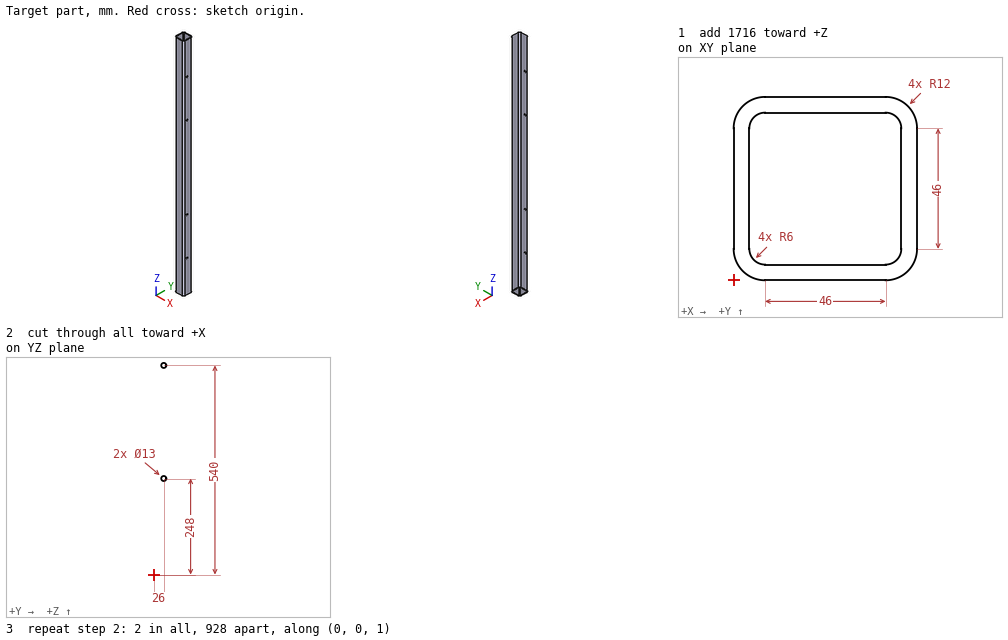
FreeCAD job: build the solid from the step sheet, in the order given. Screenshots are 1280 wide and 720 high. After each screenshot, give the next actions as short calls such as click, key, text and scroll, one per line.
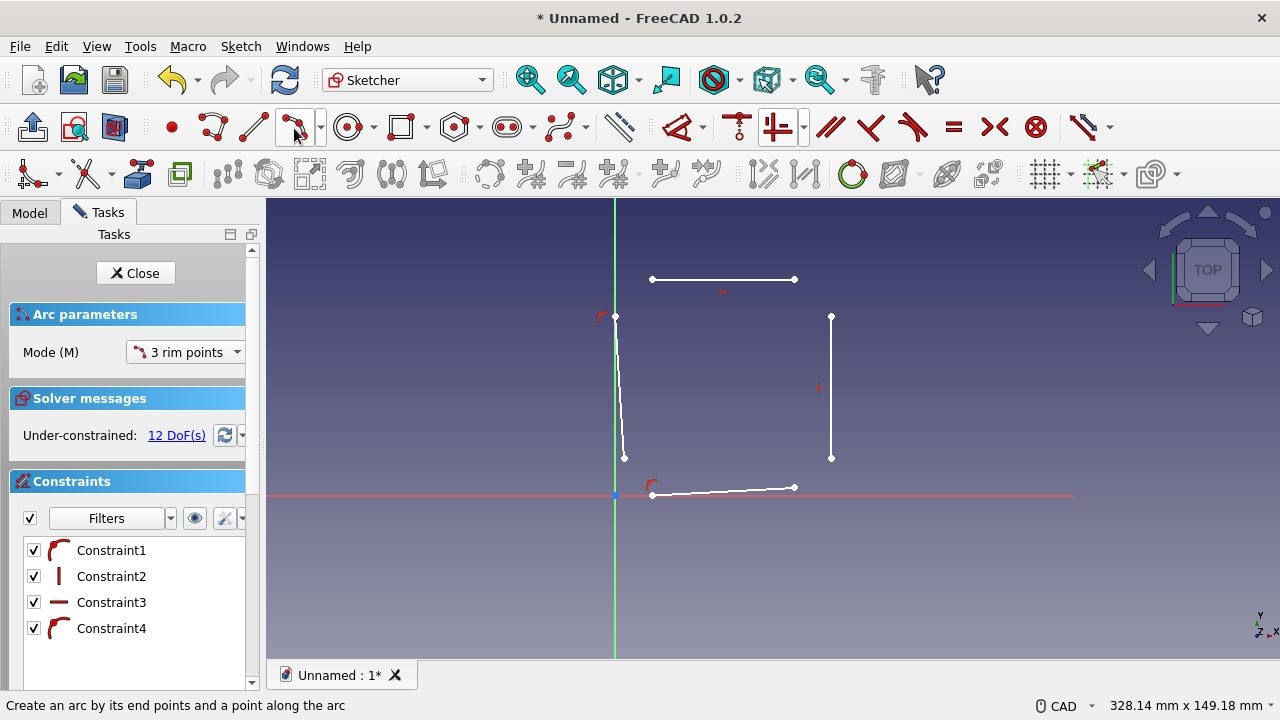
click(794, 488)
click(831, 459)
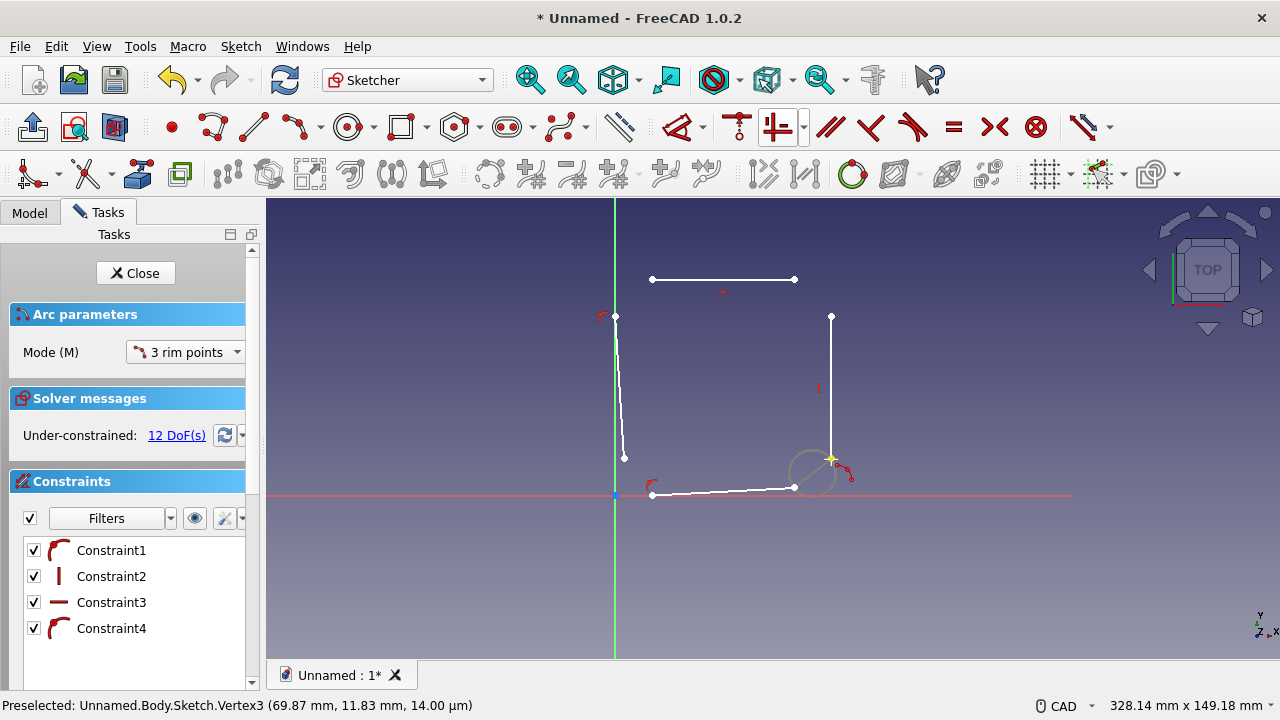
scroll(821, 485, up, 2)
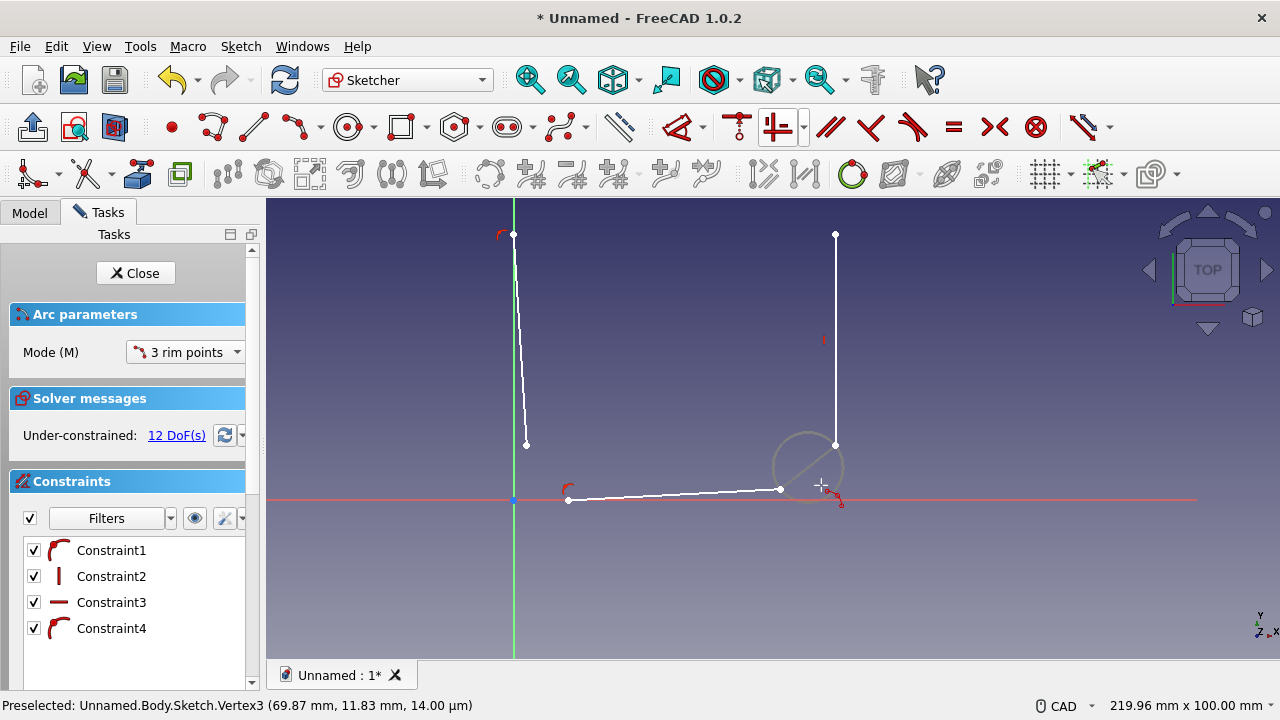
click(820, 484)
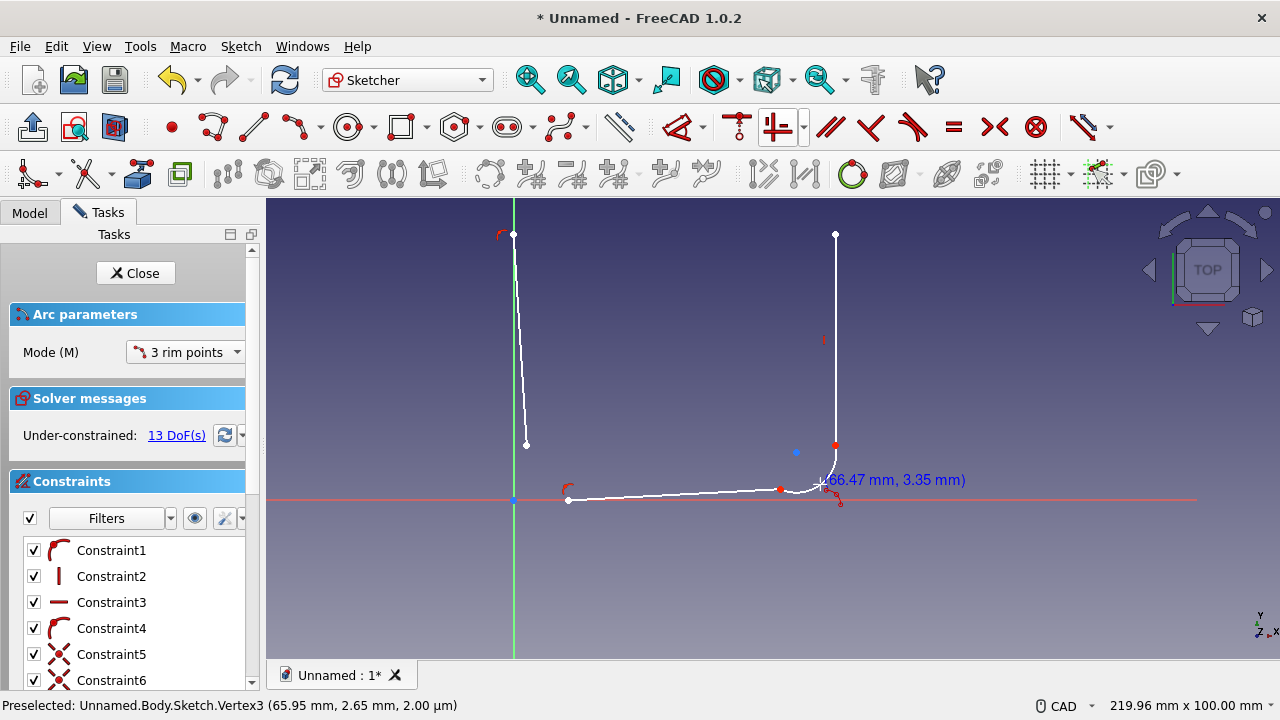
click(836, 234)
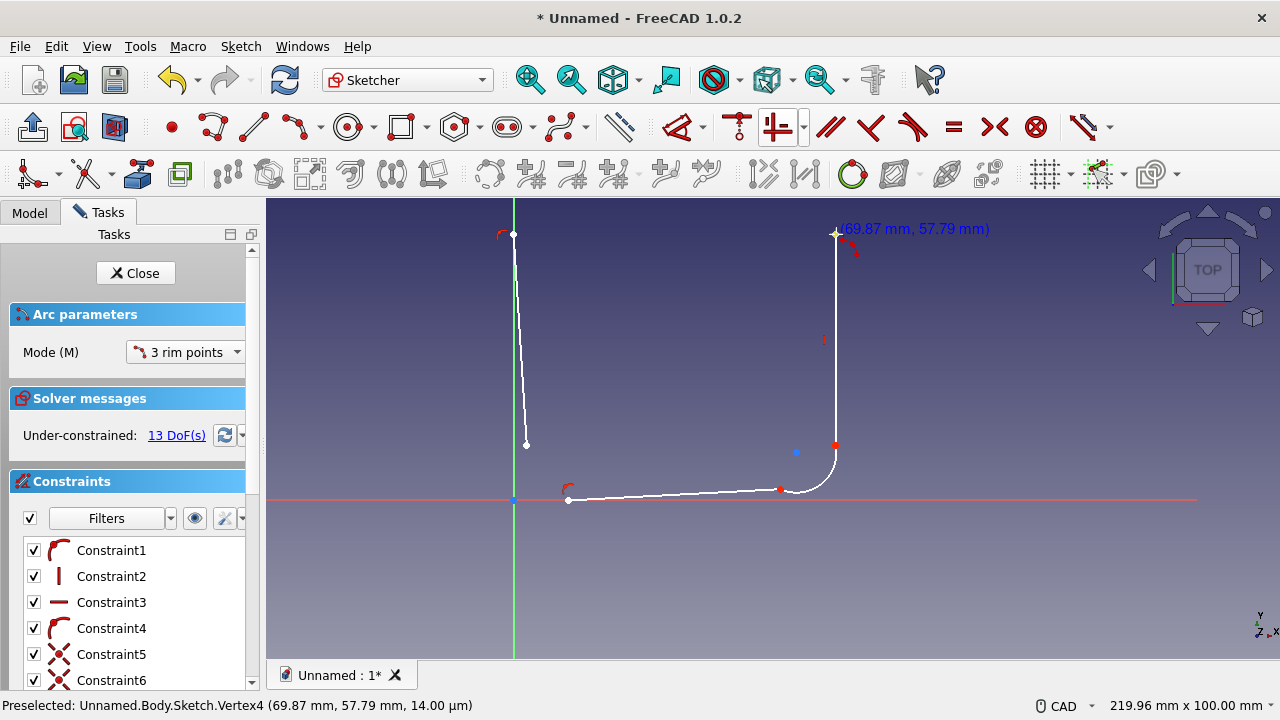
scroll(838, 631, down, 1)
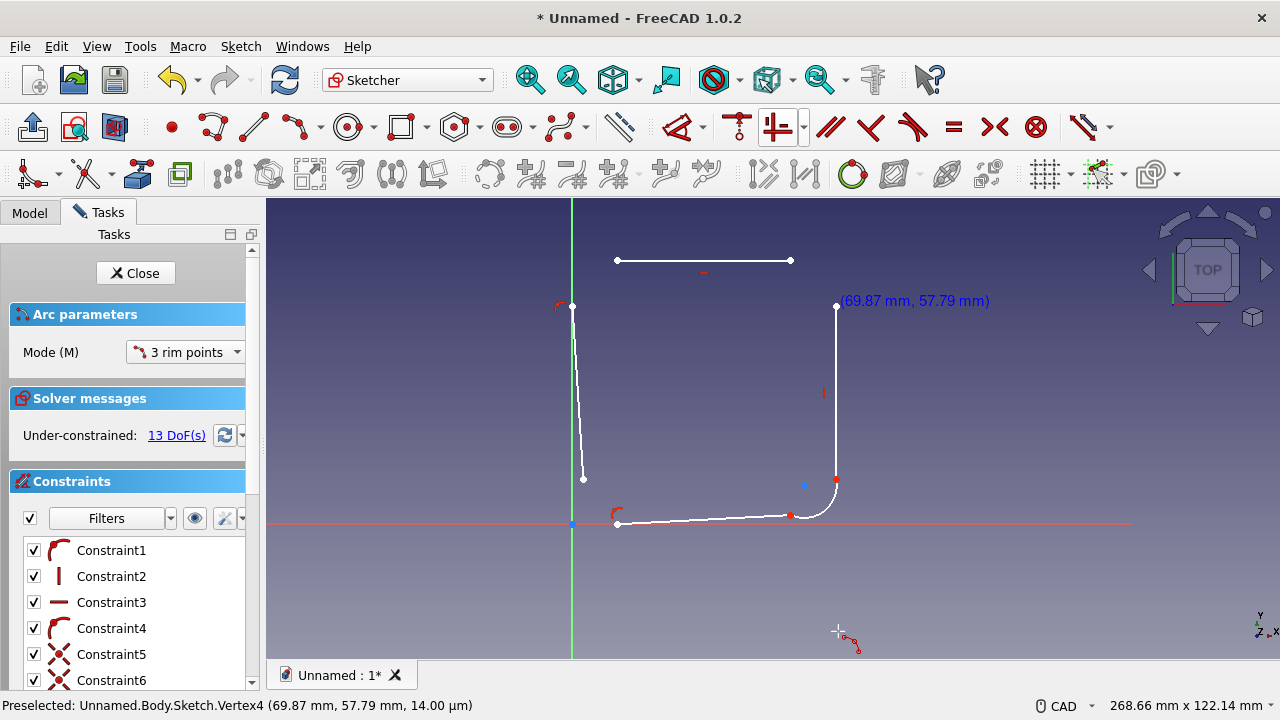
click(791, 261)
click(823, 273)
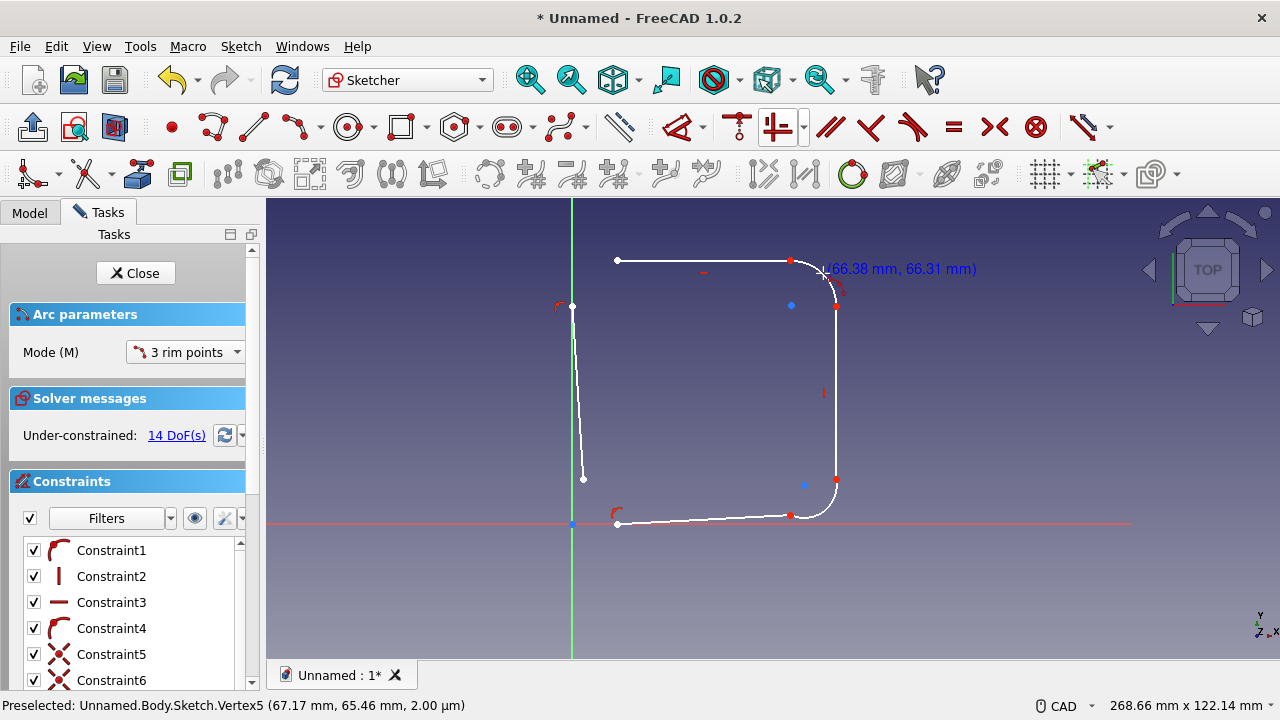
click(618, 261)
click(572, 306)
click(586, 273)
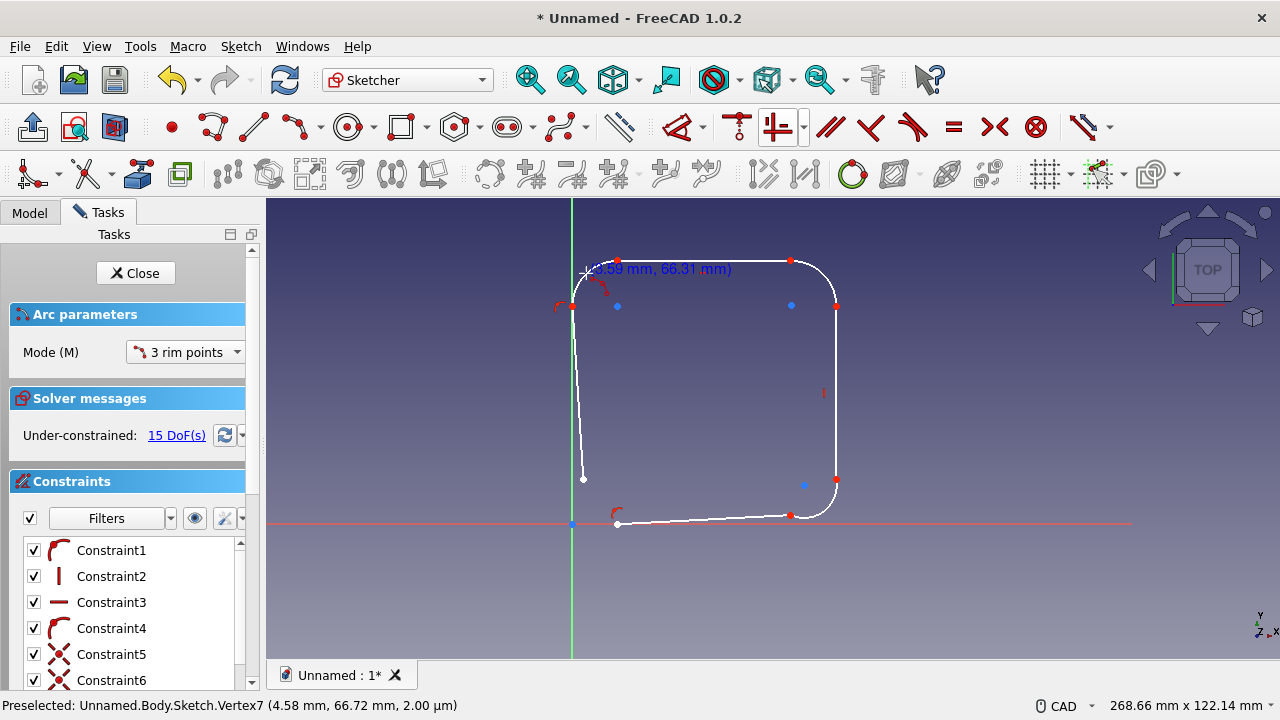
click(583, 480)
click(618, 524)
click(586, 511)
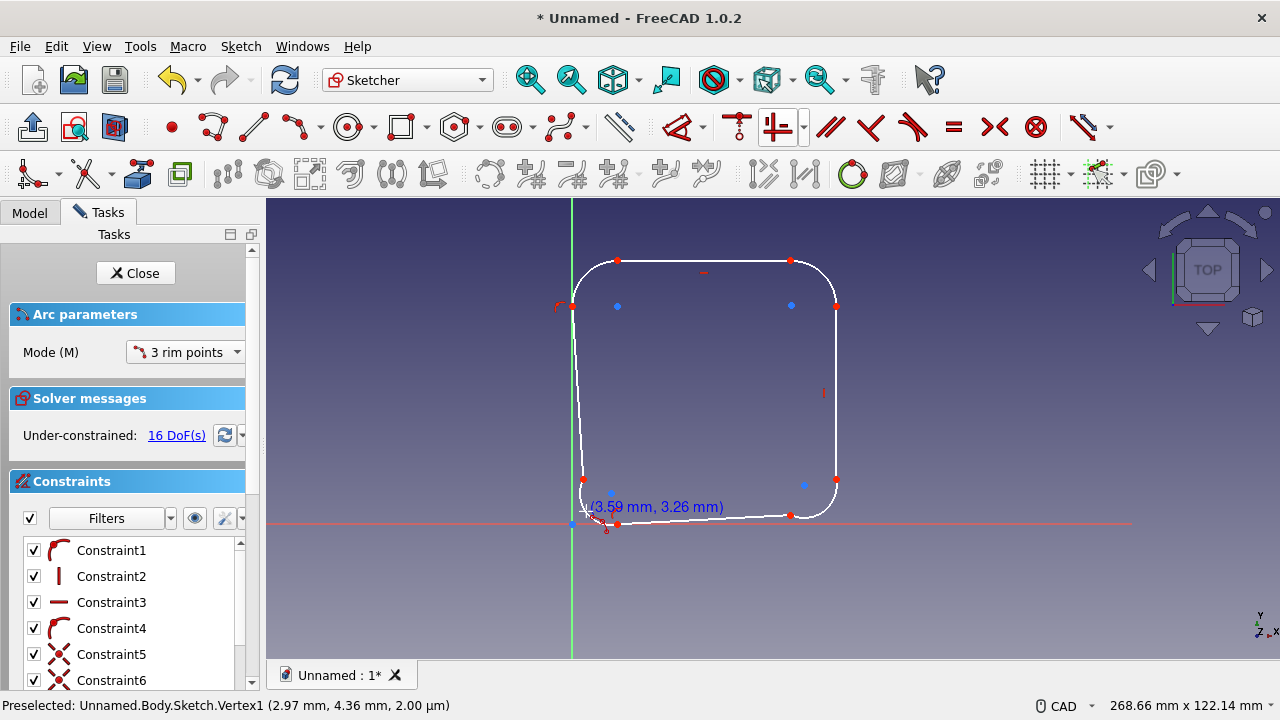
click(254, 128)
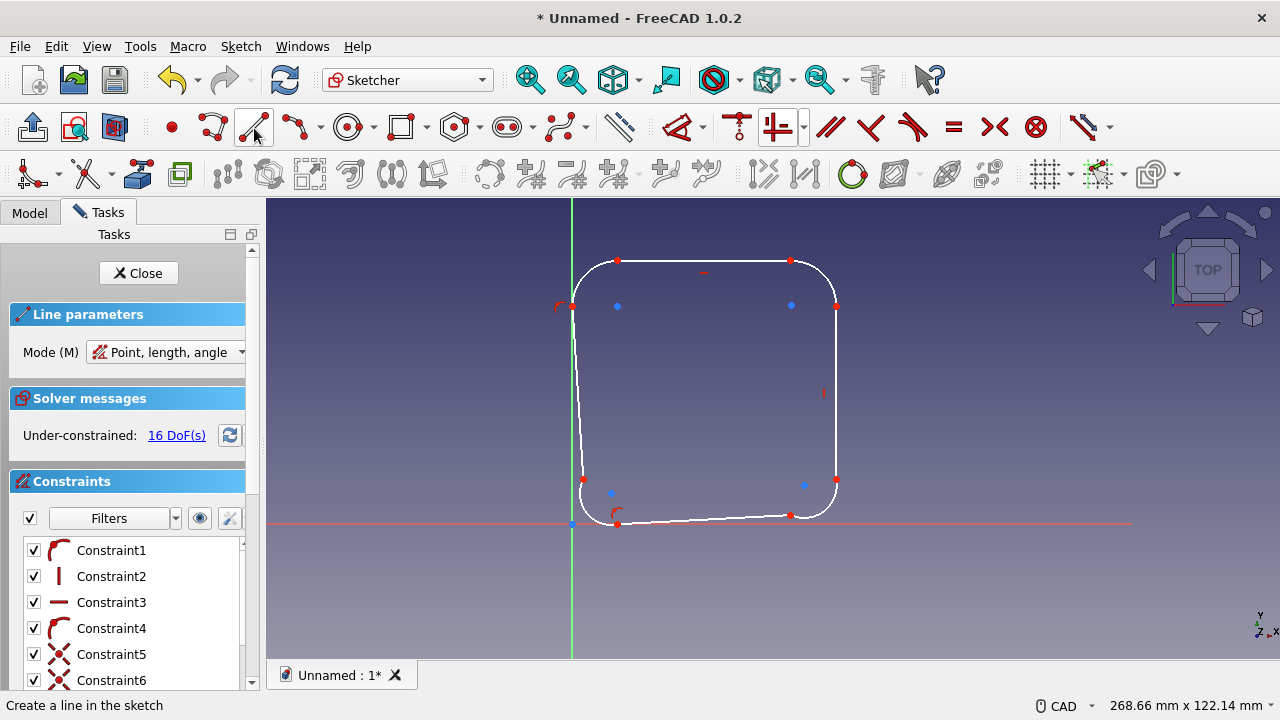
click(791, 502)
click(618, 502)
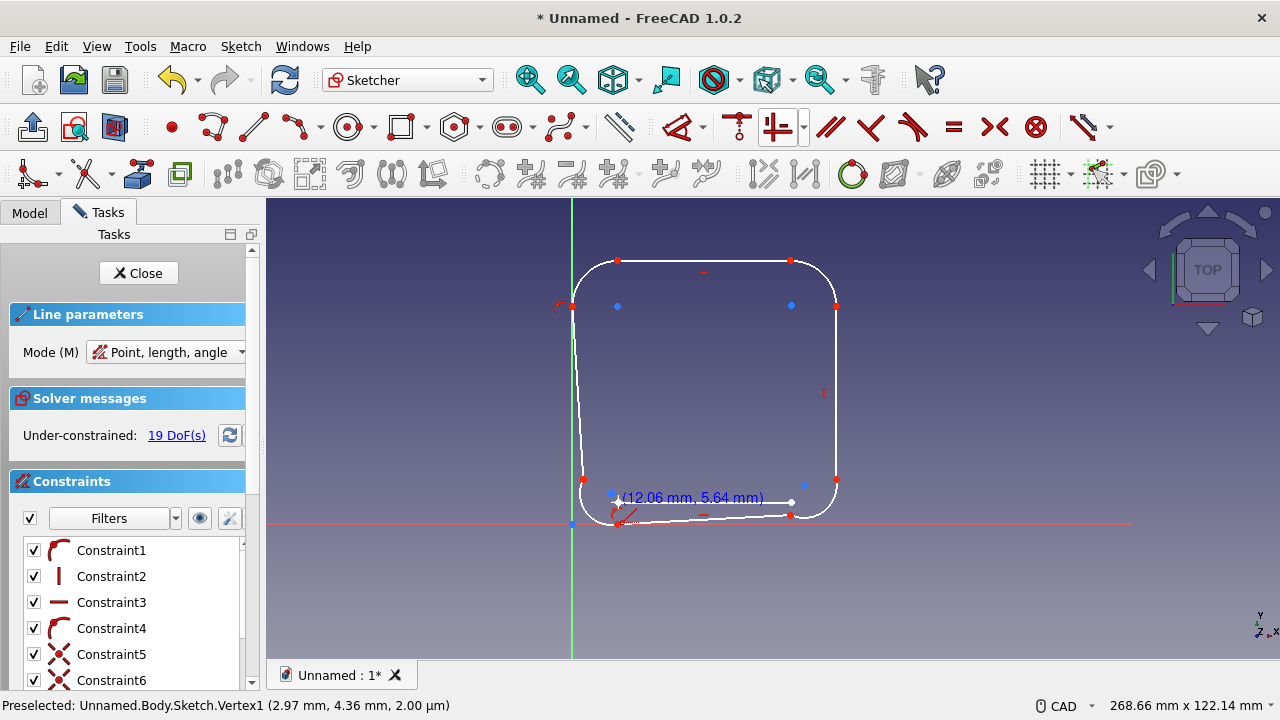
click(595, 479)
click(595, 305)